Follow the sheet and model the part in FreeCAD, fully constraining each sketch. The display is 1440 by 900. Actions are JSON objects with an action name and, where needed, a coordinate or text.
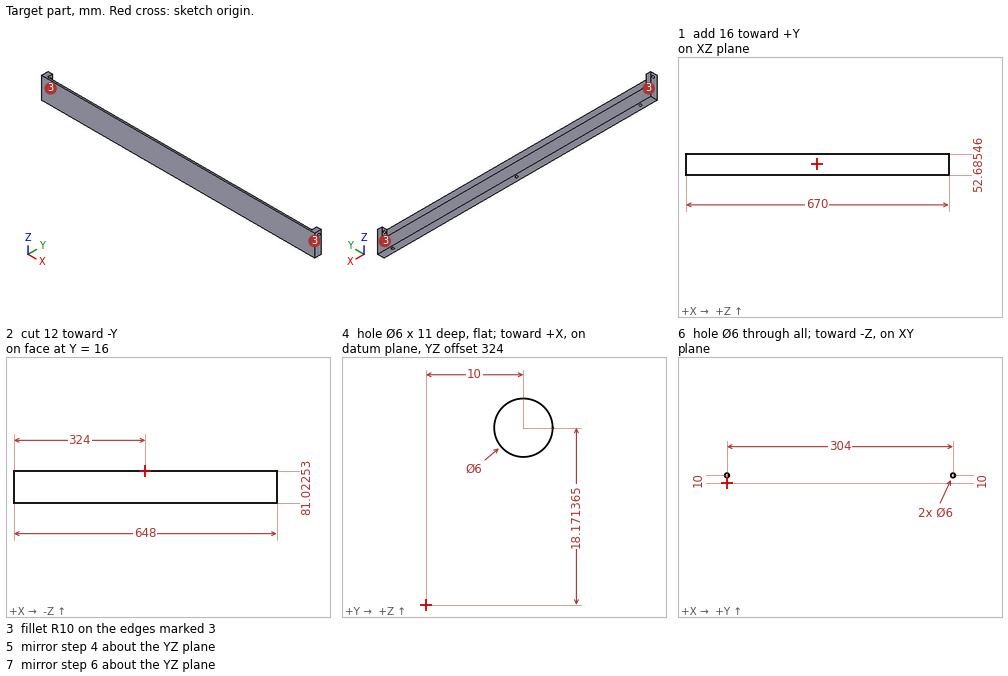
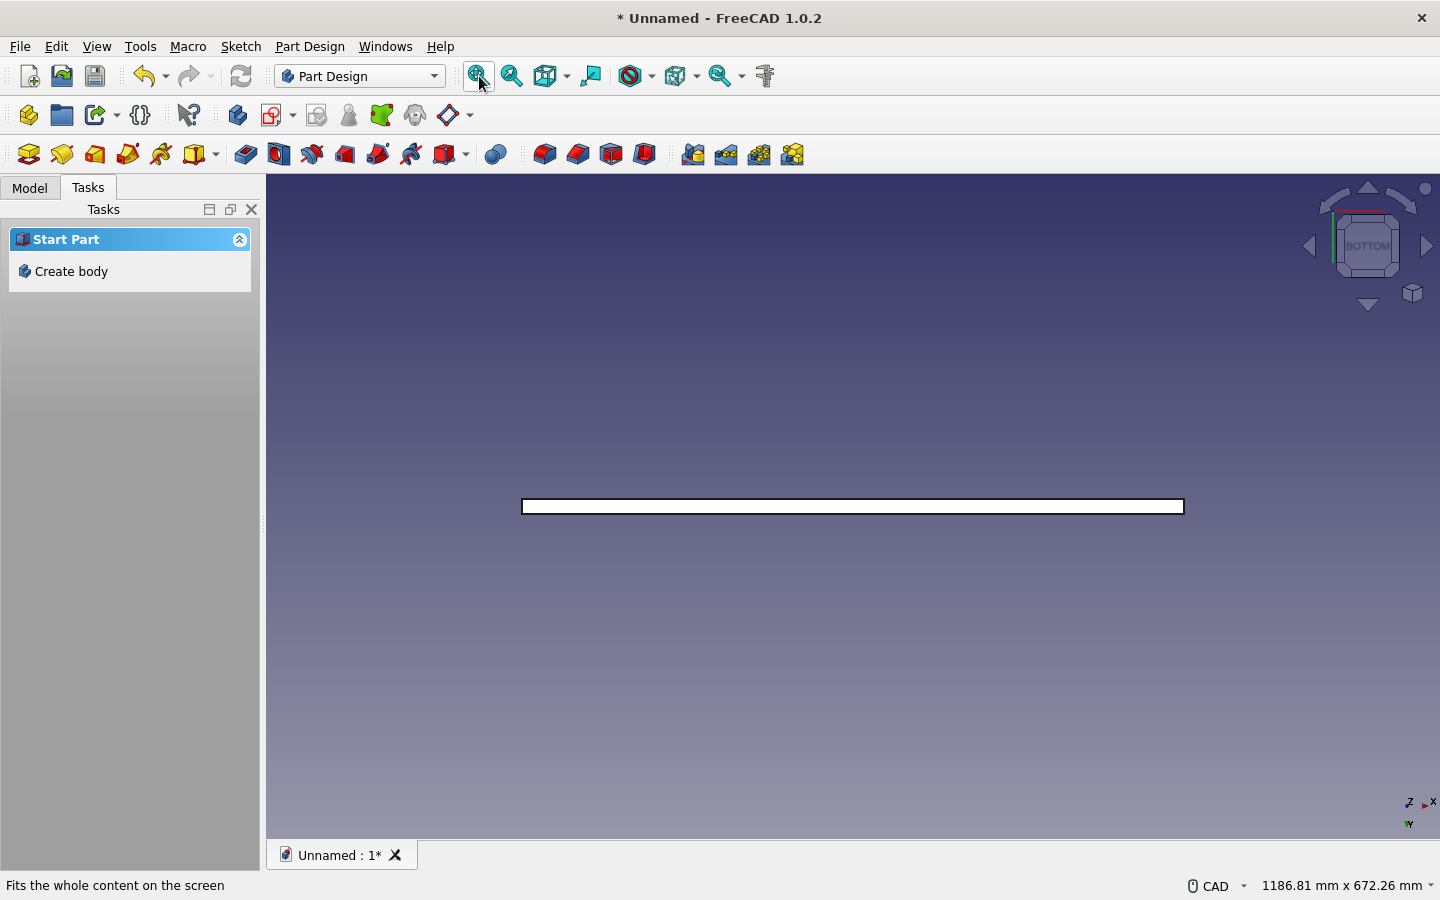
{"action": "key", "text": "4"}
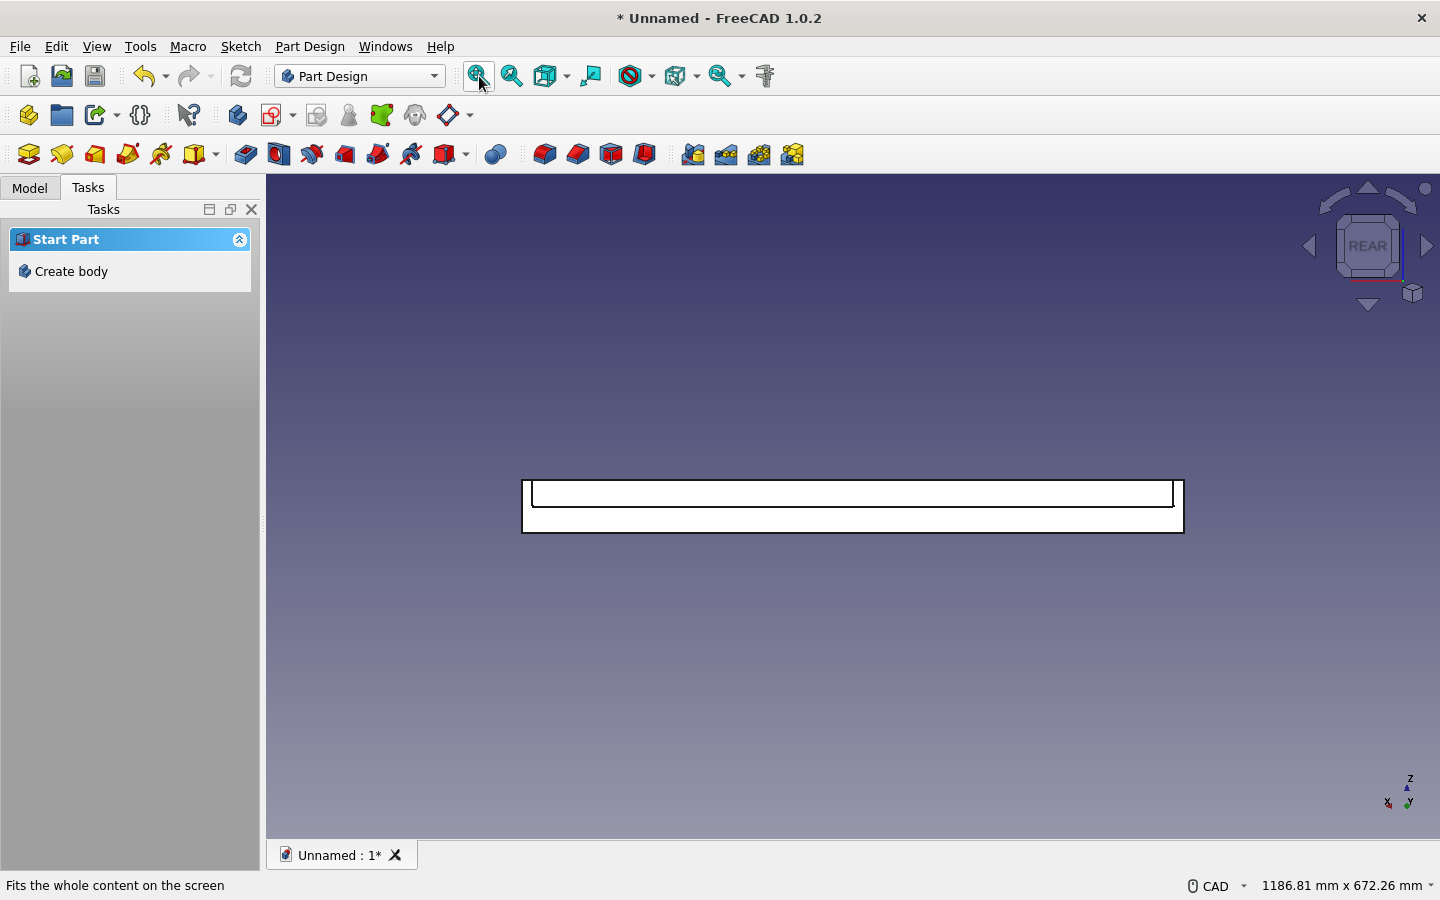
{"action": "scroll", "coordinate": [532, 506], "scroll_direction": "up", "scroll_amount": 7}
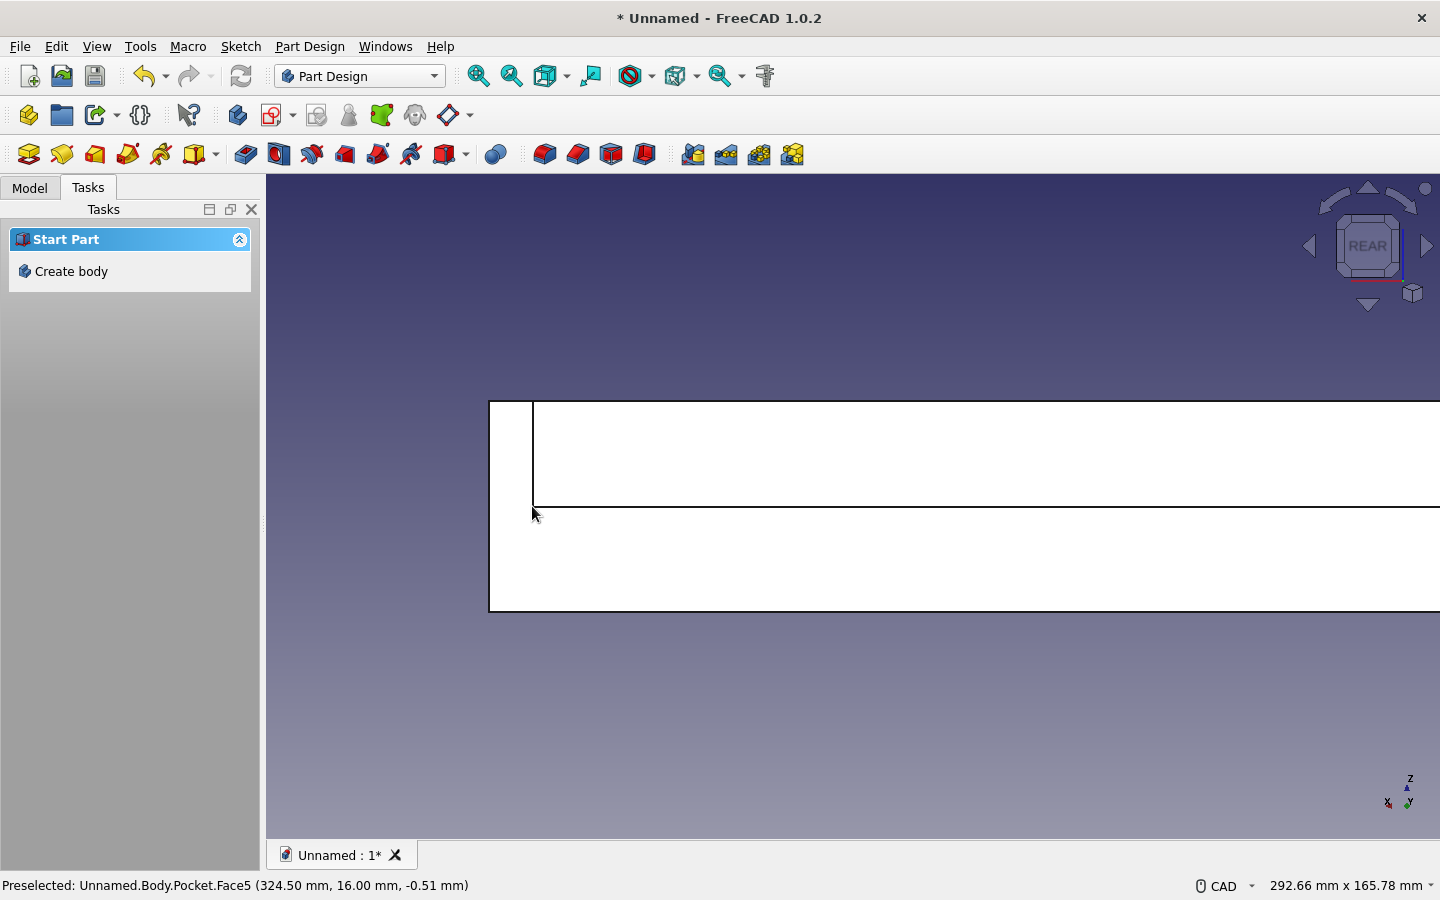
{"action": "key", "text": "v f"}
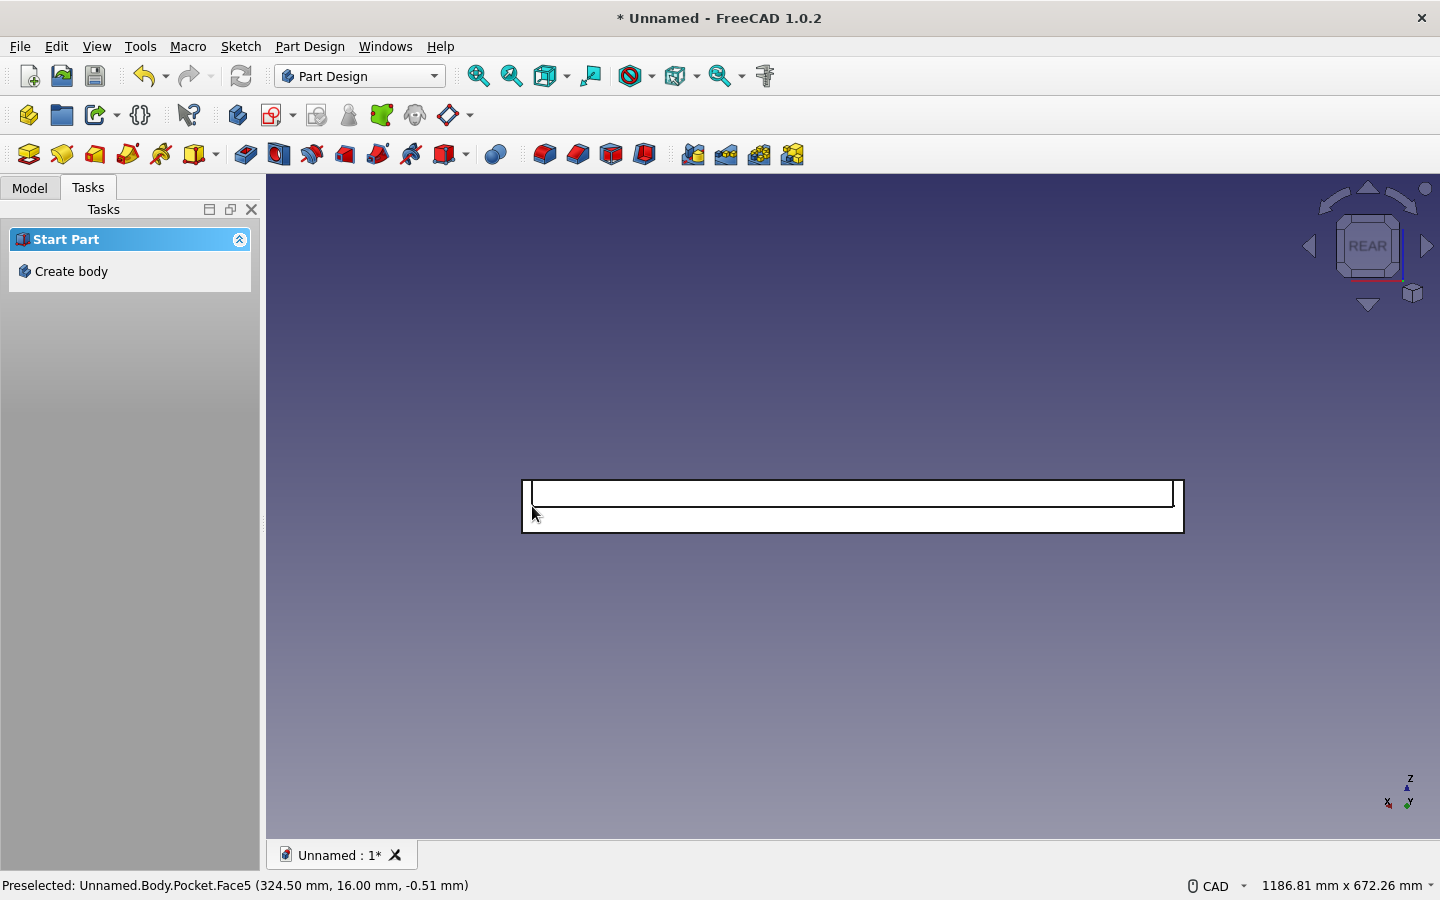
{"action": "key", "text": "6"}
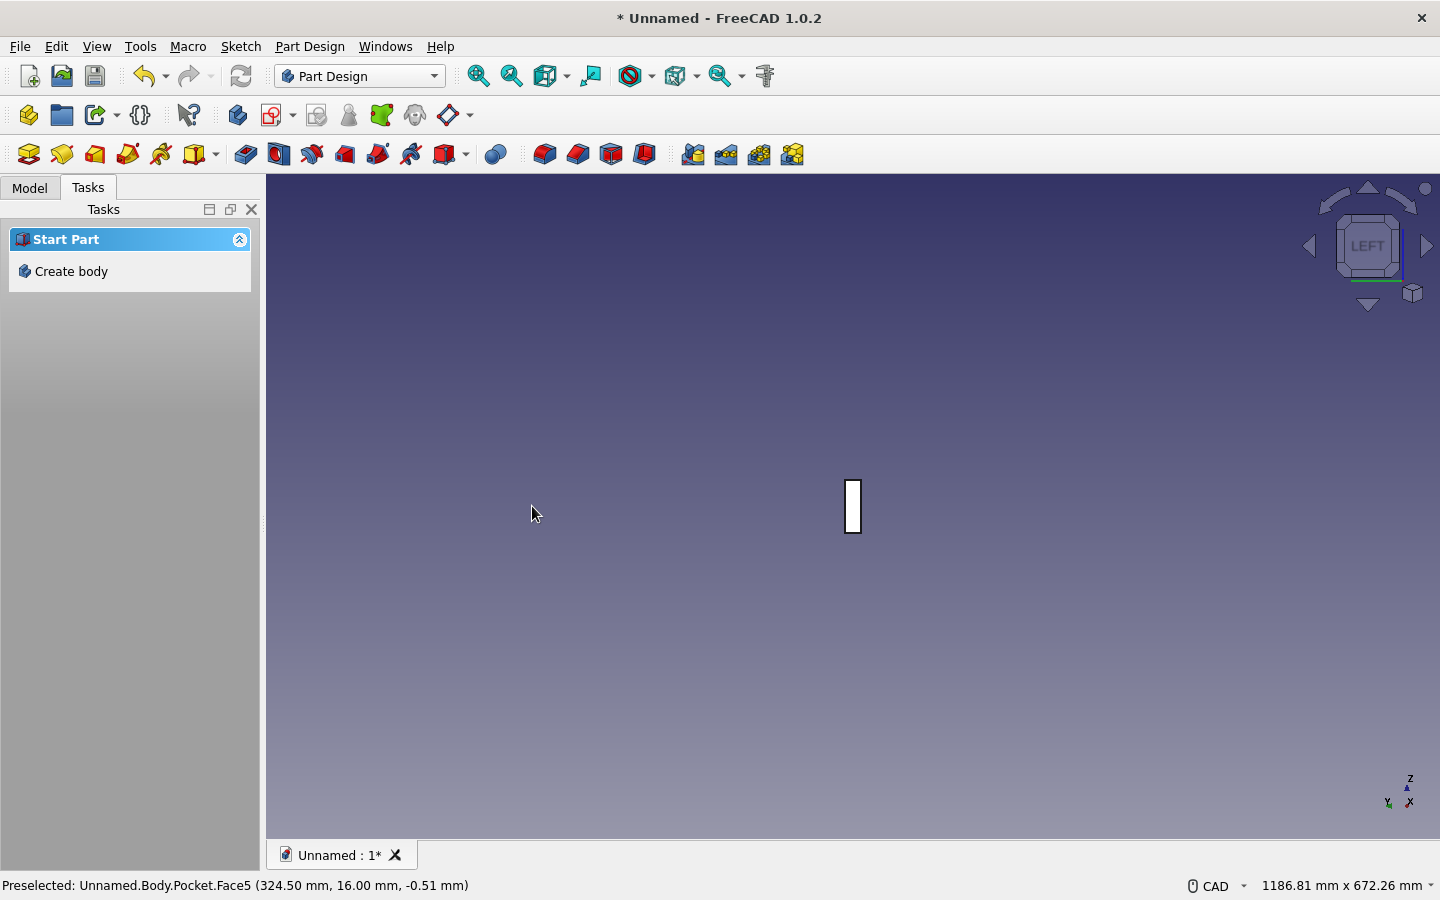
{"action": "left_click", "coordinate": [479, 76]}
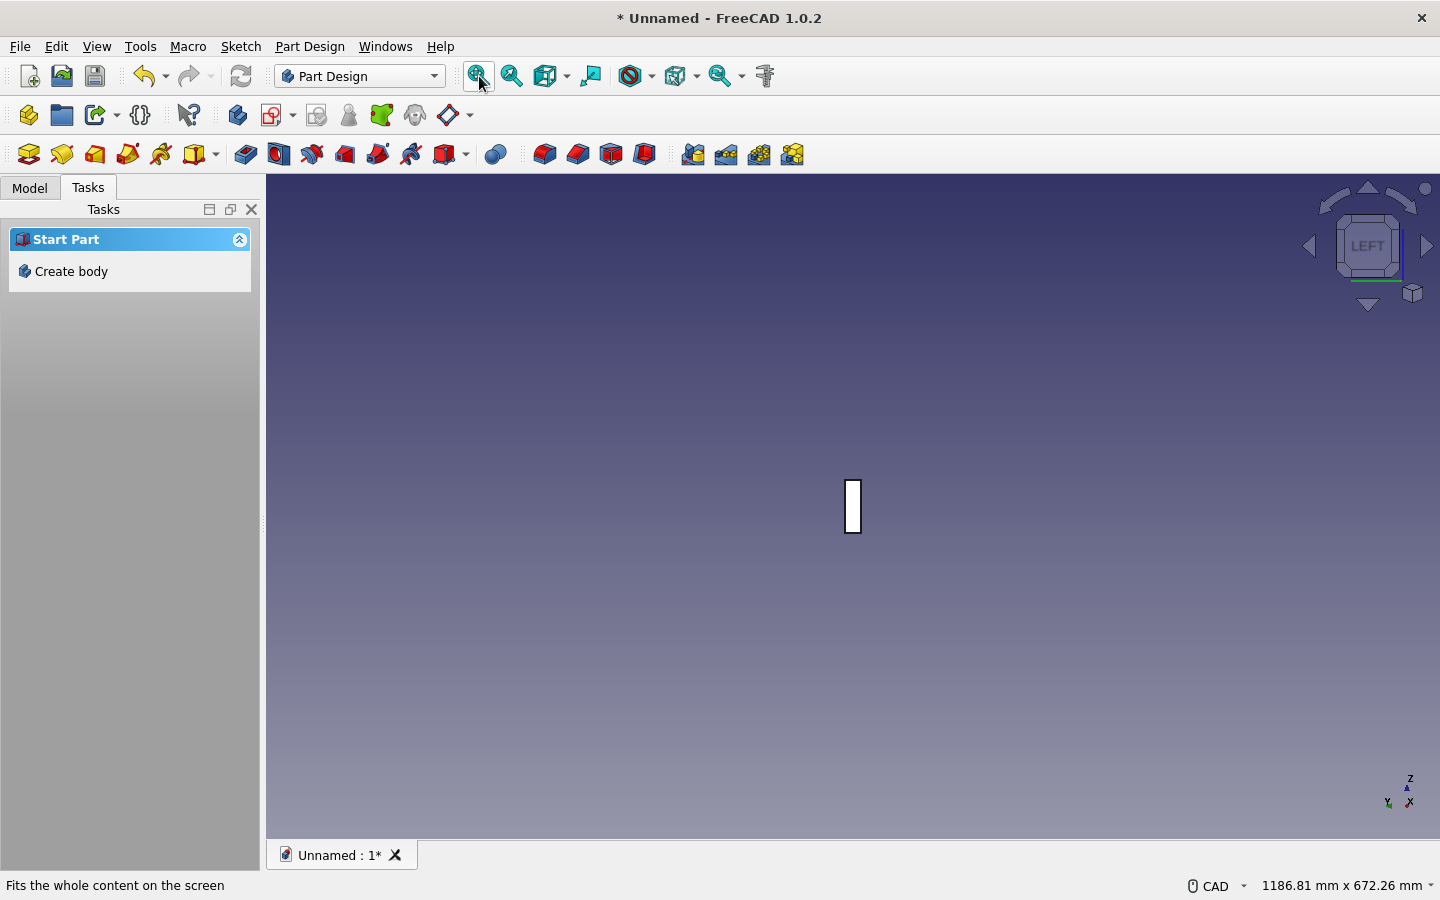
{"action": "scroll", "coordinate": [851, 505], "scroll_direction": "up", "scroll_amount": 7}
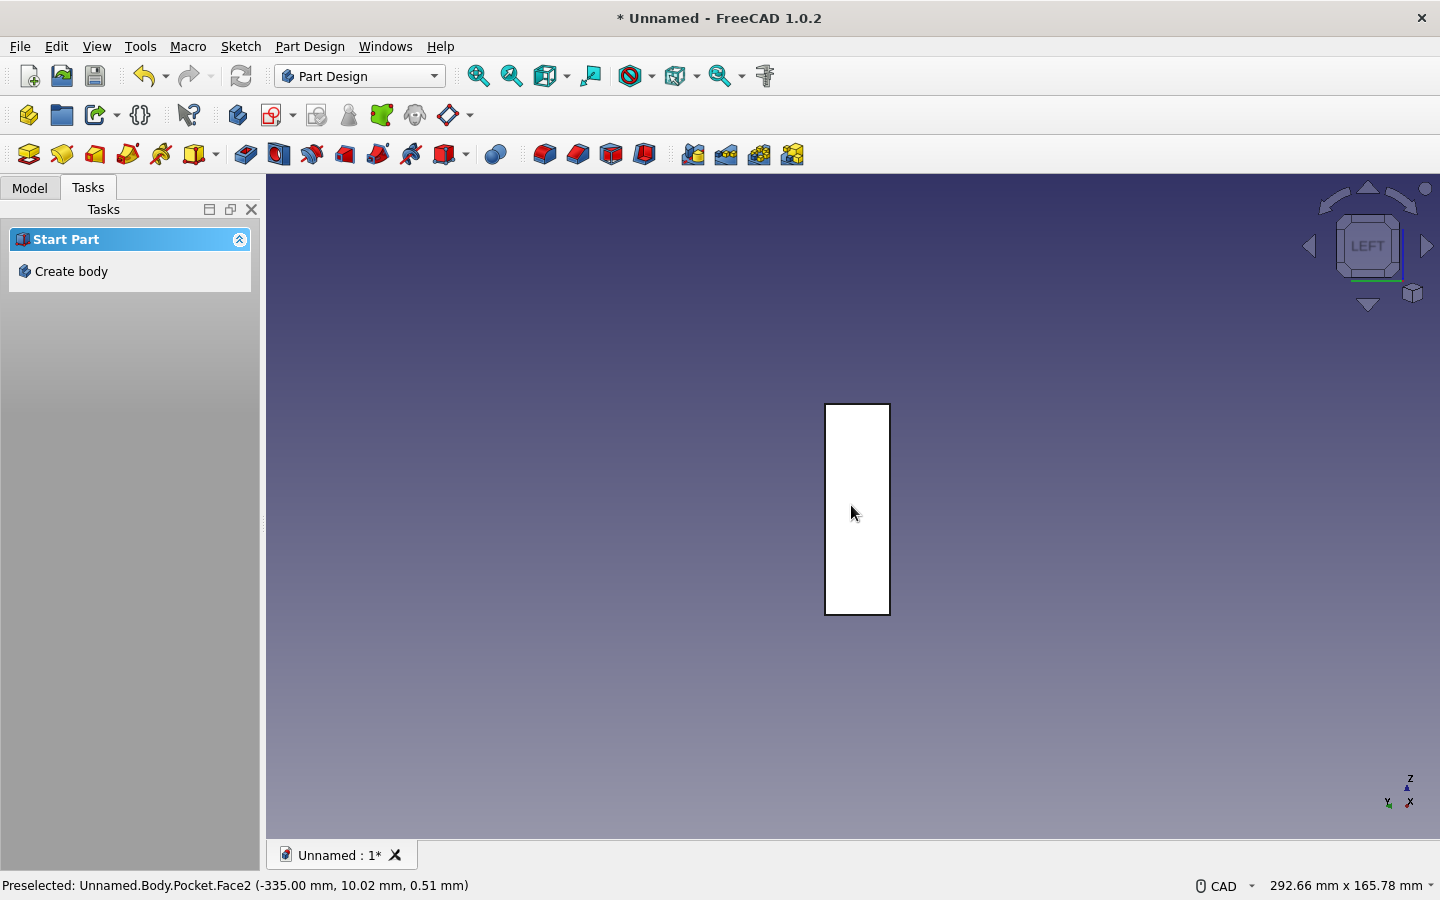
{"action": "left_click", "coordinate": [479, 76]}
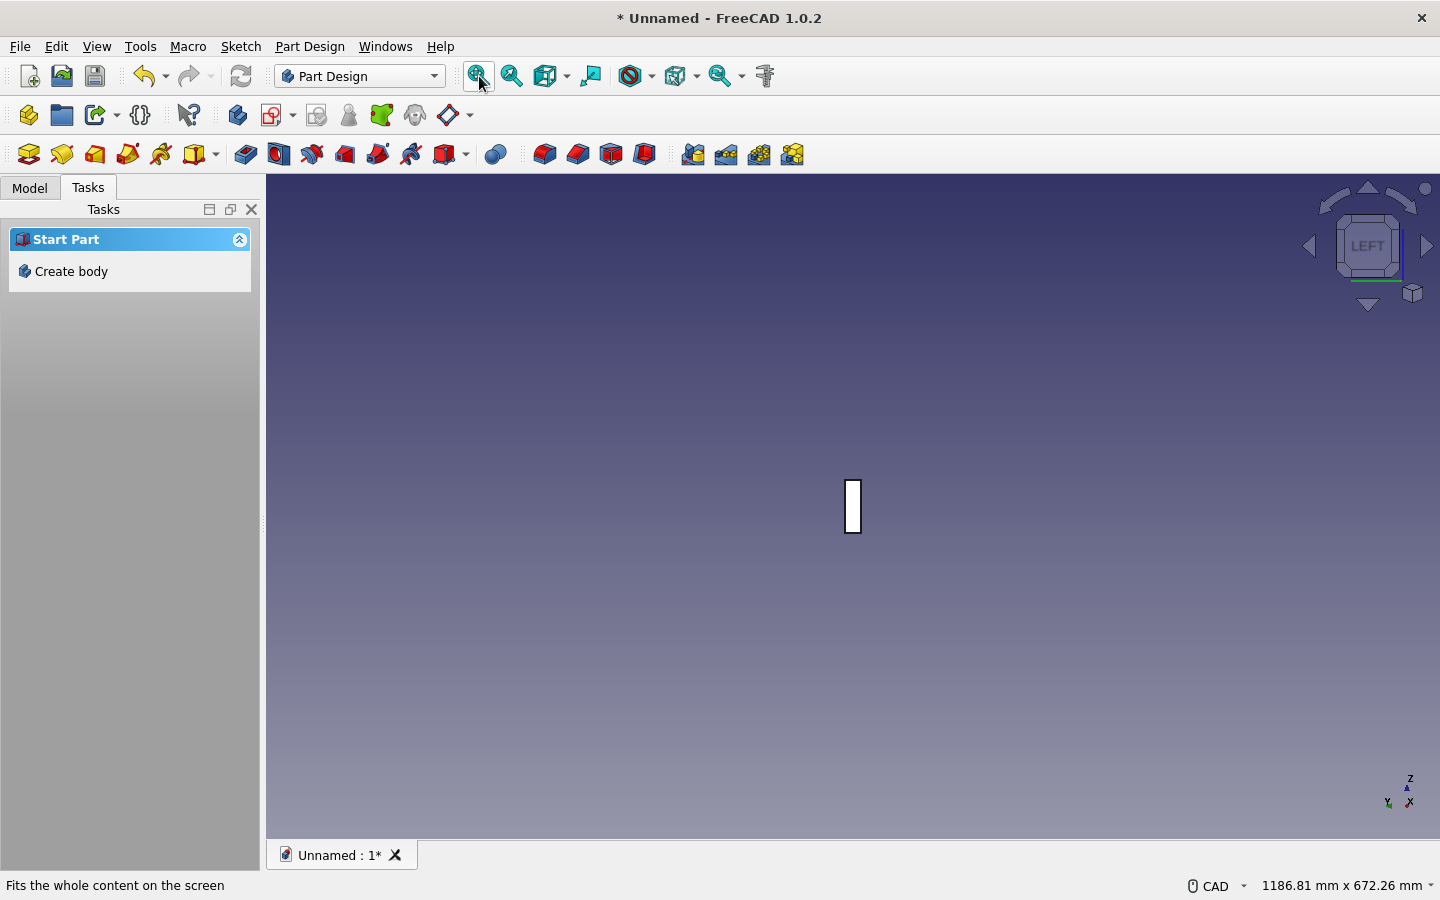
{"action": "key", "text": "v 3"}